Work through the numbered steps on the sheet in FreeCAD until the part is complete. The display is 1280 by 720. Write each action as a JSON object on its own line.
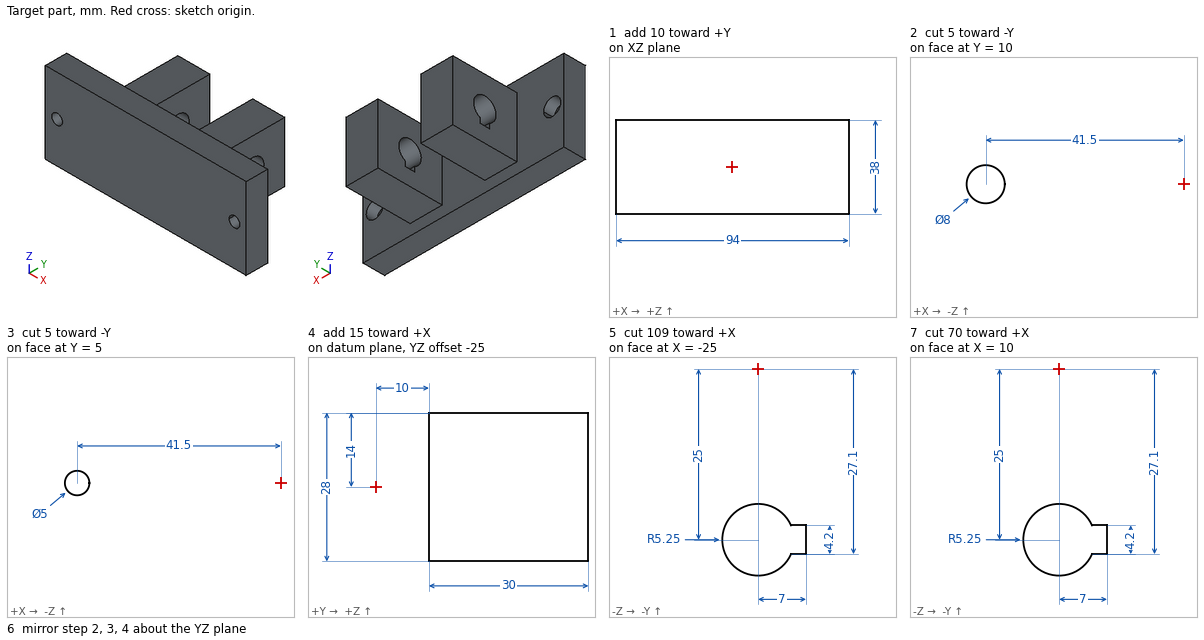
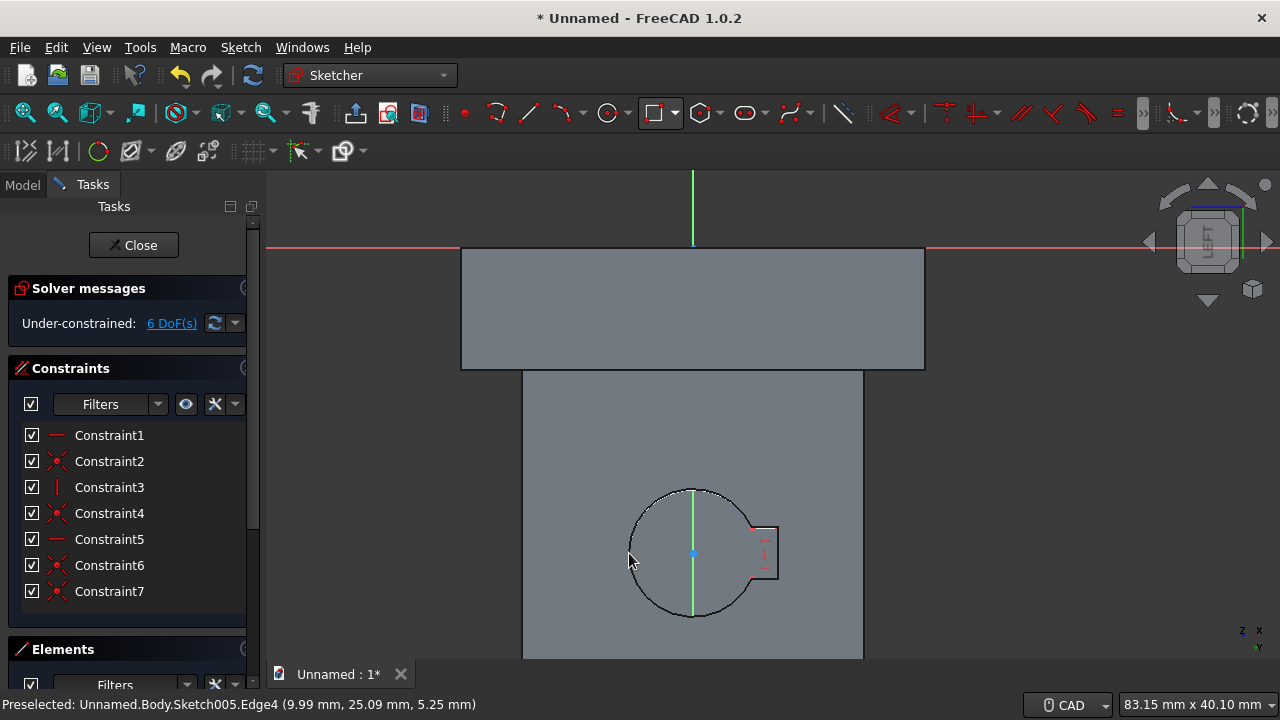
{"action": "left_click", "coordinate": [693, 554]}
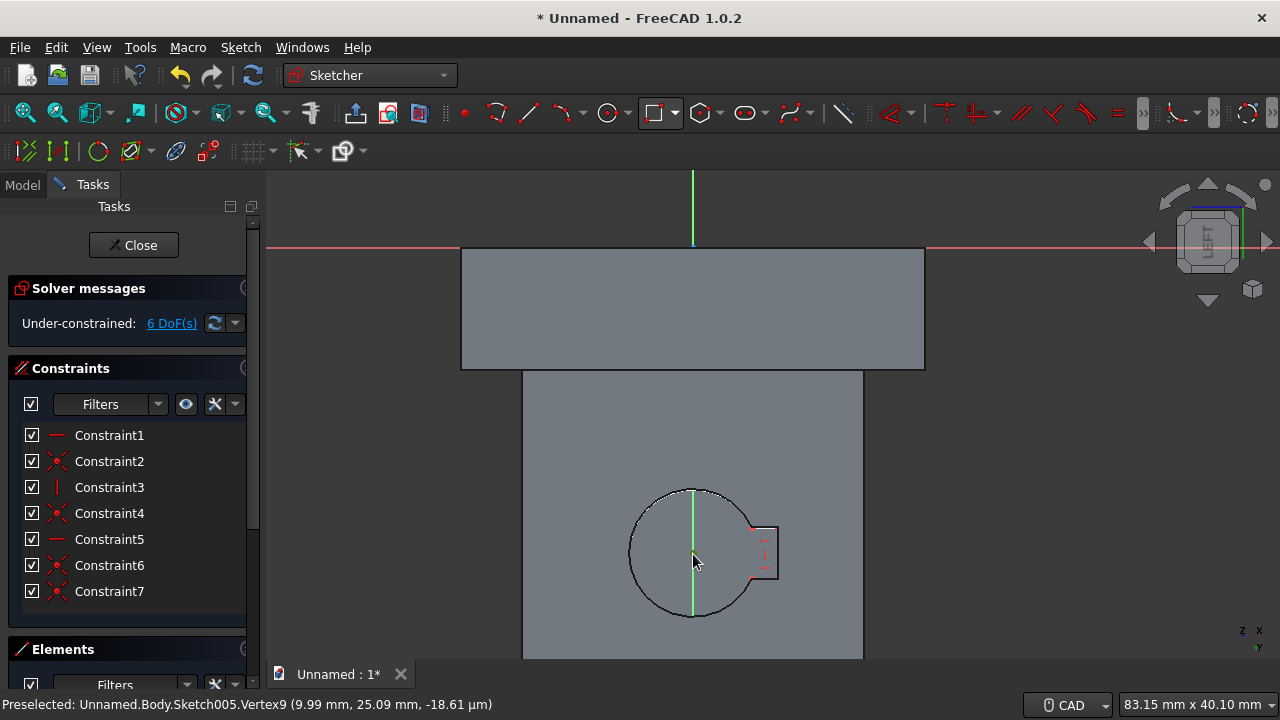
{"action": "left_click", "coordinate": [693, 569]}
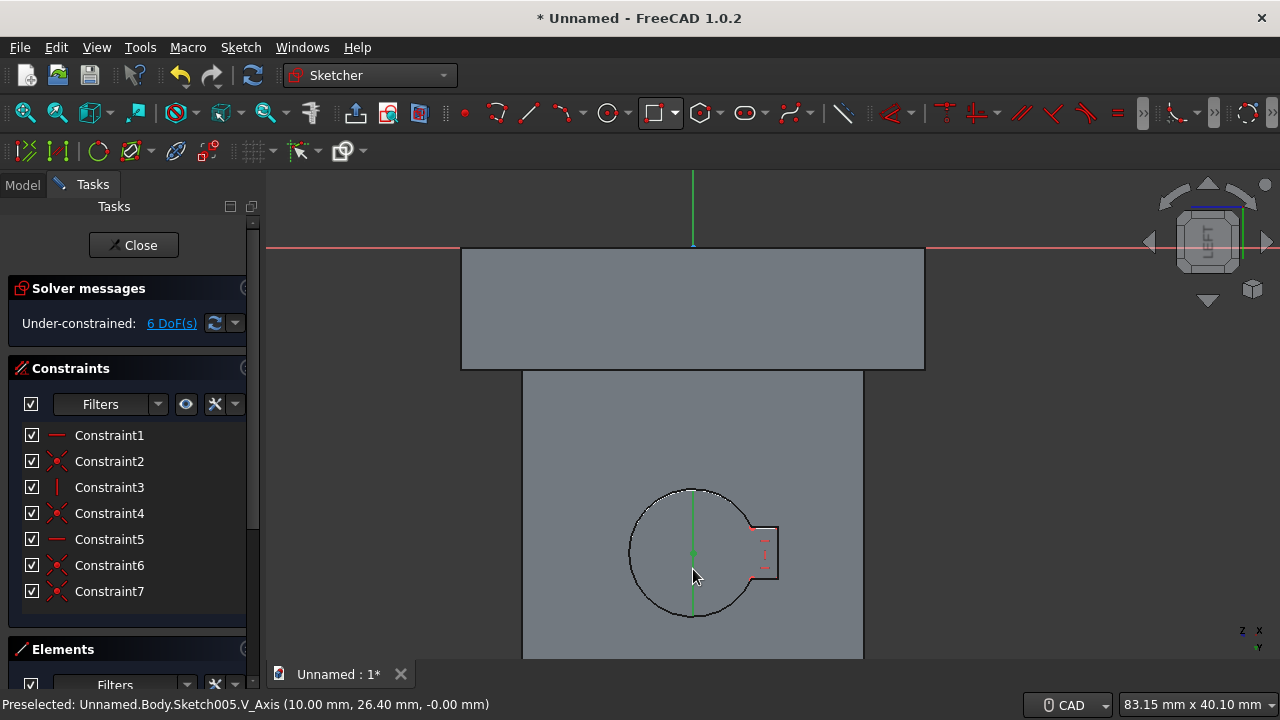
{"action": "left_click", "coordinate": [946, 114]}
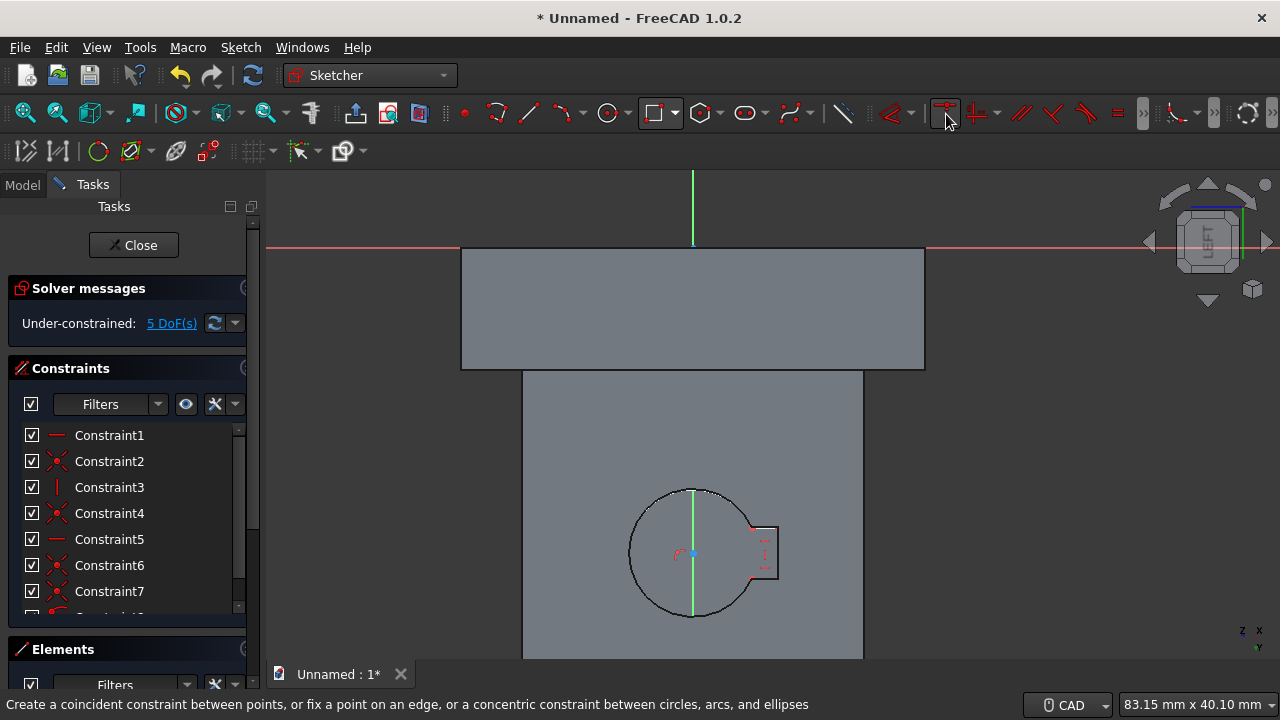
{"action": "left_click", "coordinate": [890, 114]}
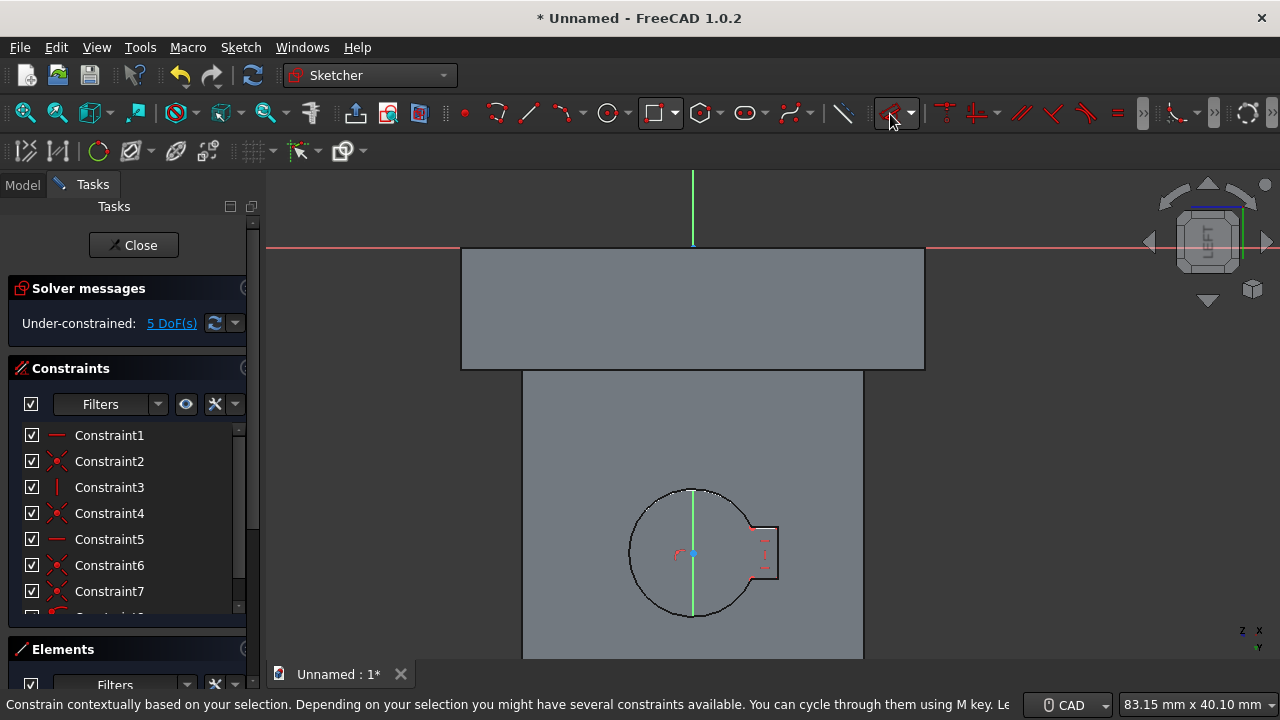
{"action": "left_click", "coordinate": [663, 497]}
{"action": "left_click", "coordinate": [648, 469]}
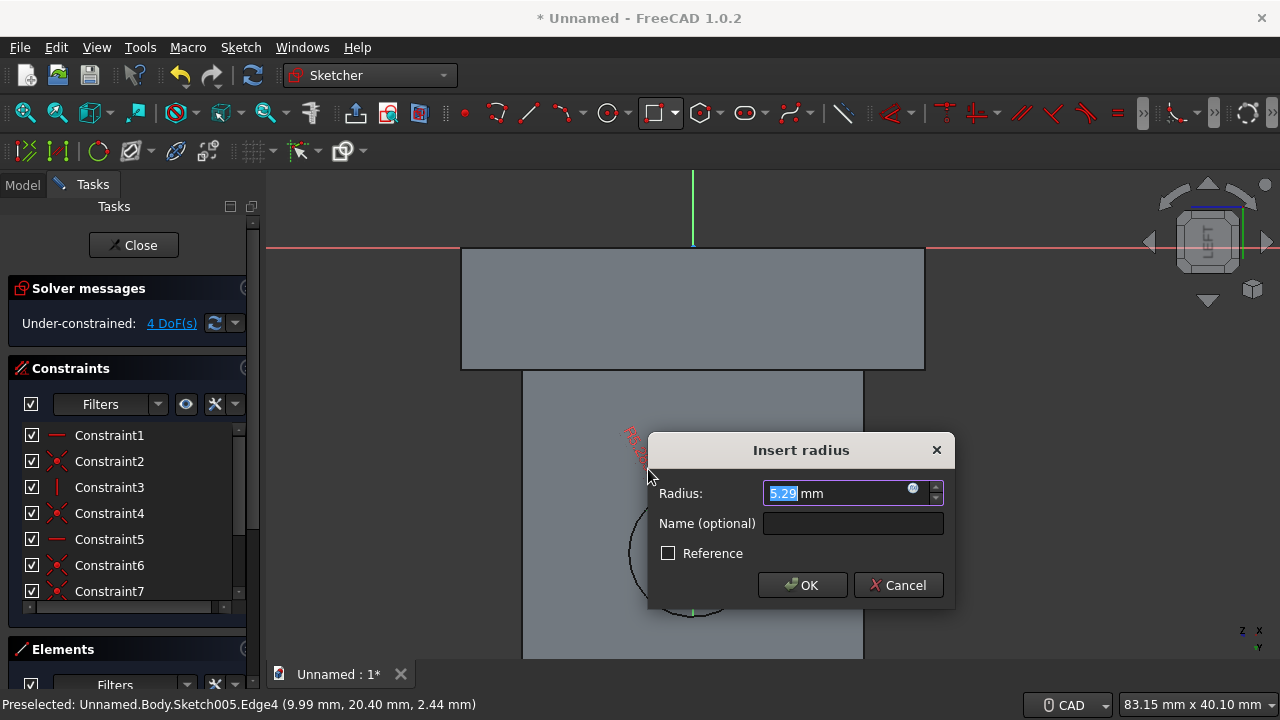
{"action": "type", "text": "5.25"}
{"action": "key", "text": "Return"}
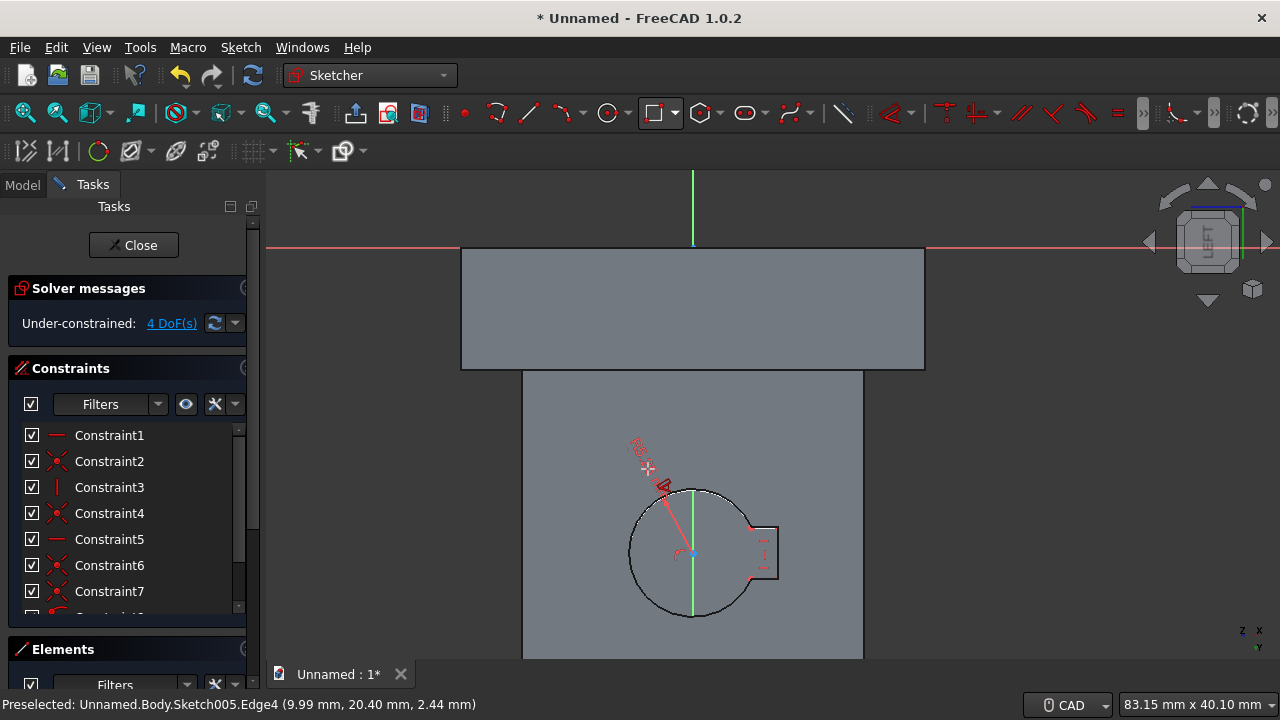
{"action": "left_click", "coordinate": [778, 580]}
{"action": "left_click", "coordinate": [755, 614]}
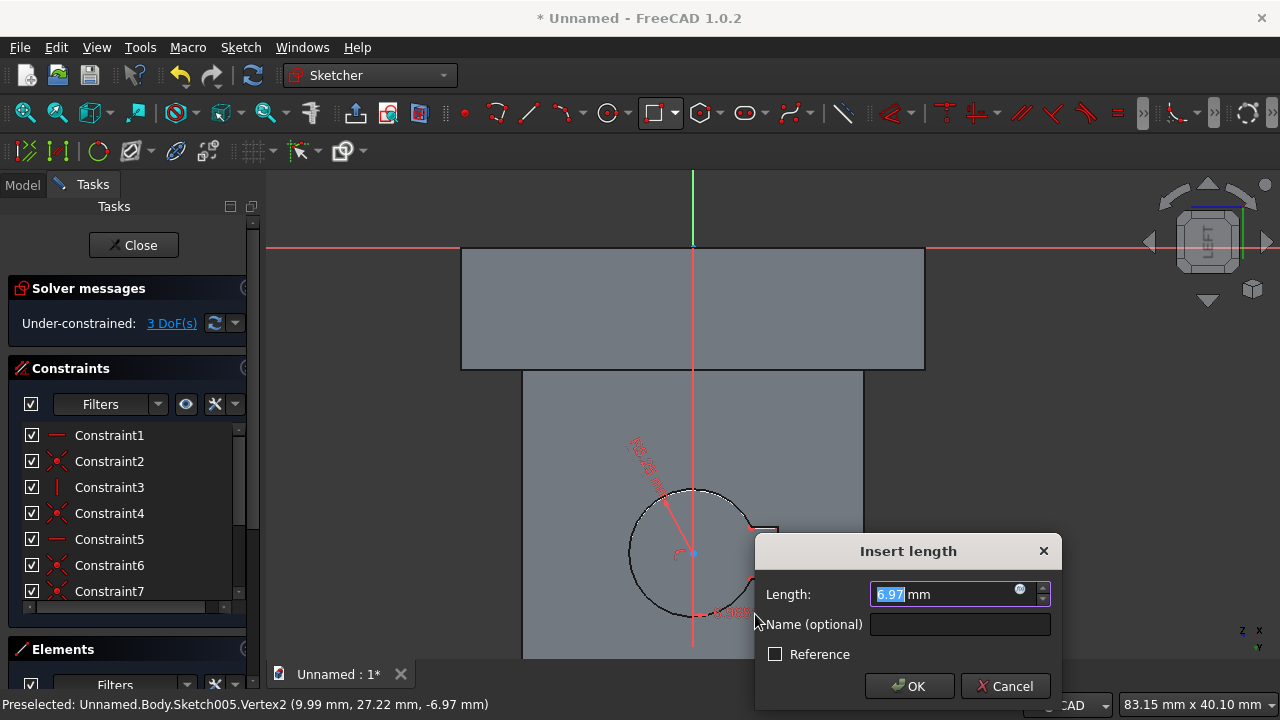
{"action": "type", "text": "7"}
{"action": "key", "text": "Return"}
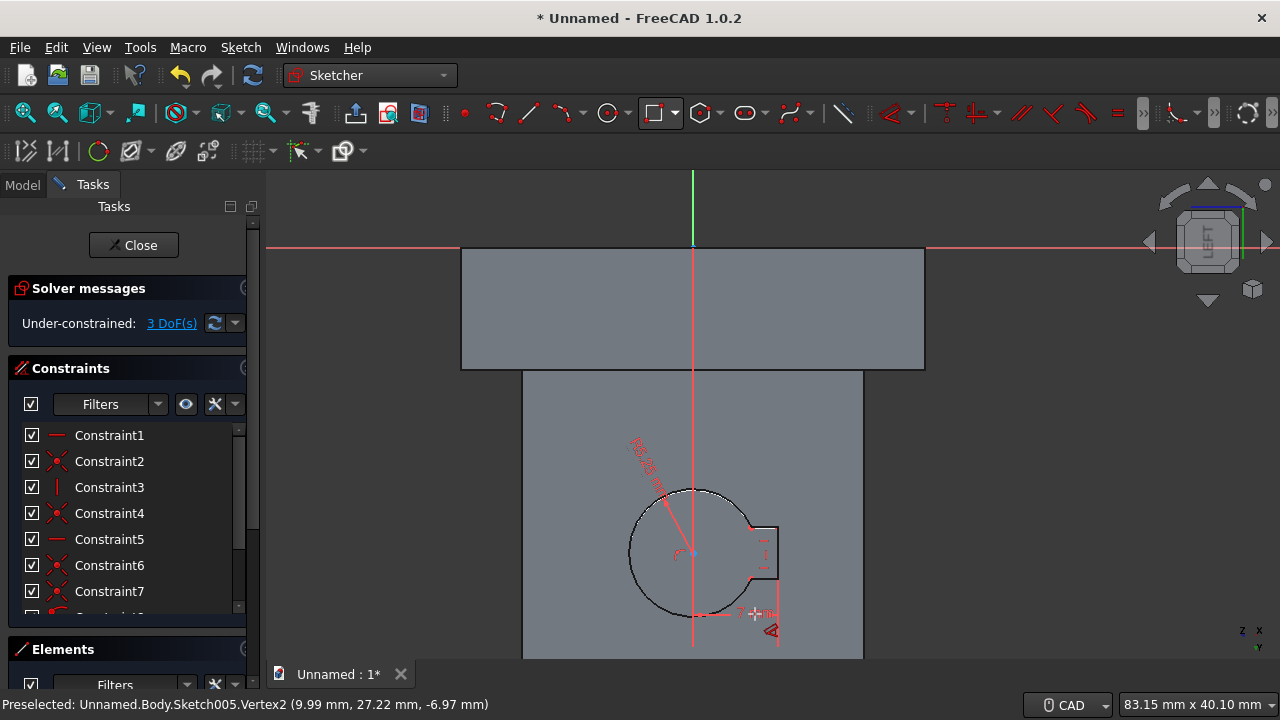
{"action": "left_click", "coordinate": [778, 564]}
{"action": "left_click", "coordinate": [812, 554]}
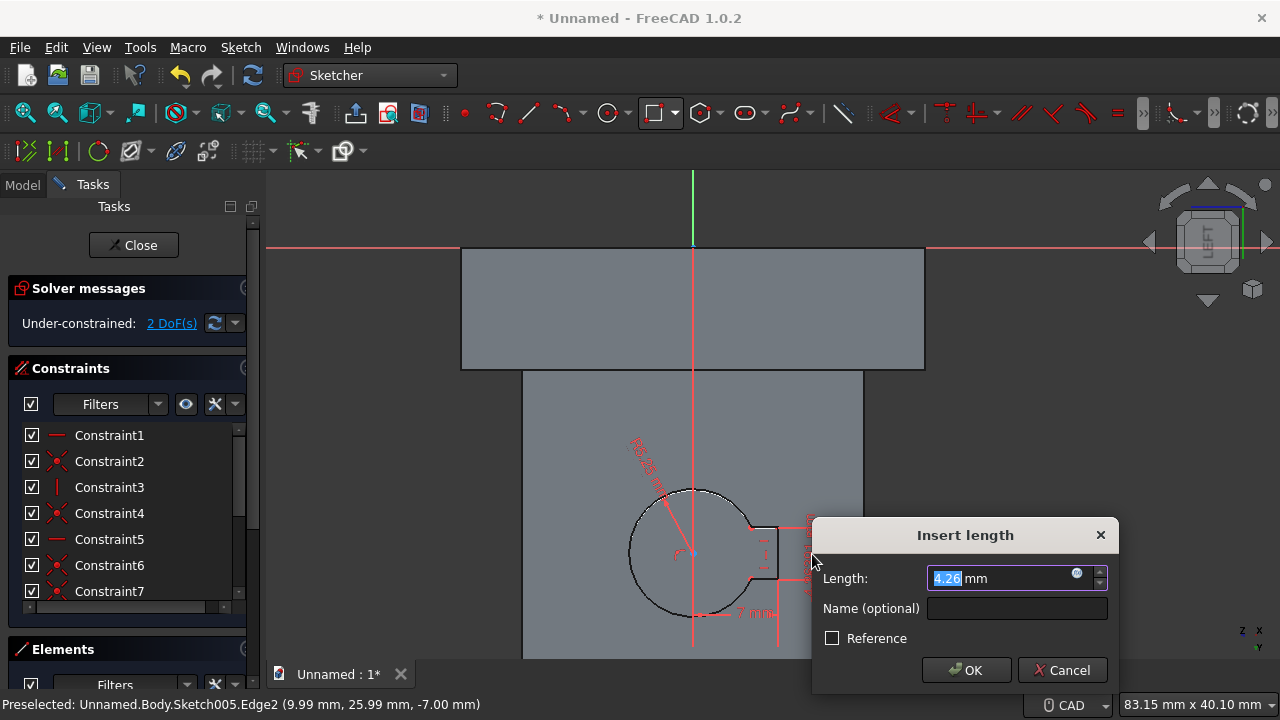
{"action": "type", "text": "4.2"}
{"action": "key", "text": "Return"}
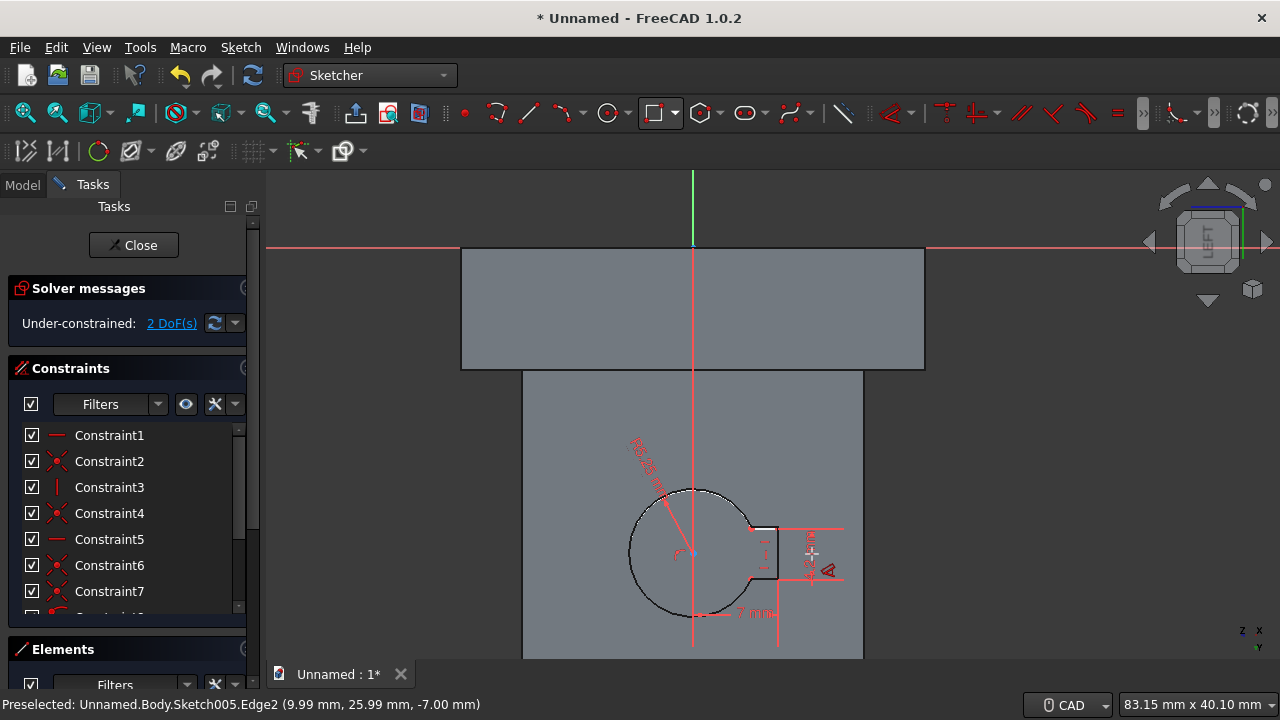
{"action": "left_click", "coordinate": [693, 554]}
{"action": "left_click", "coordinate": [659, 401]}